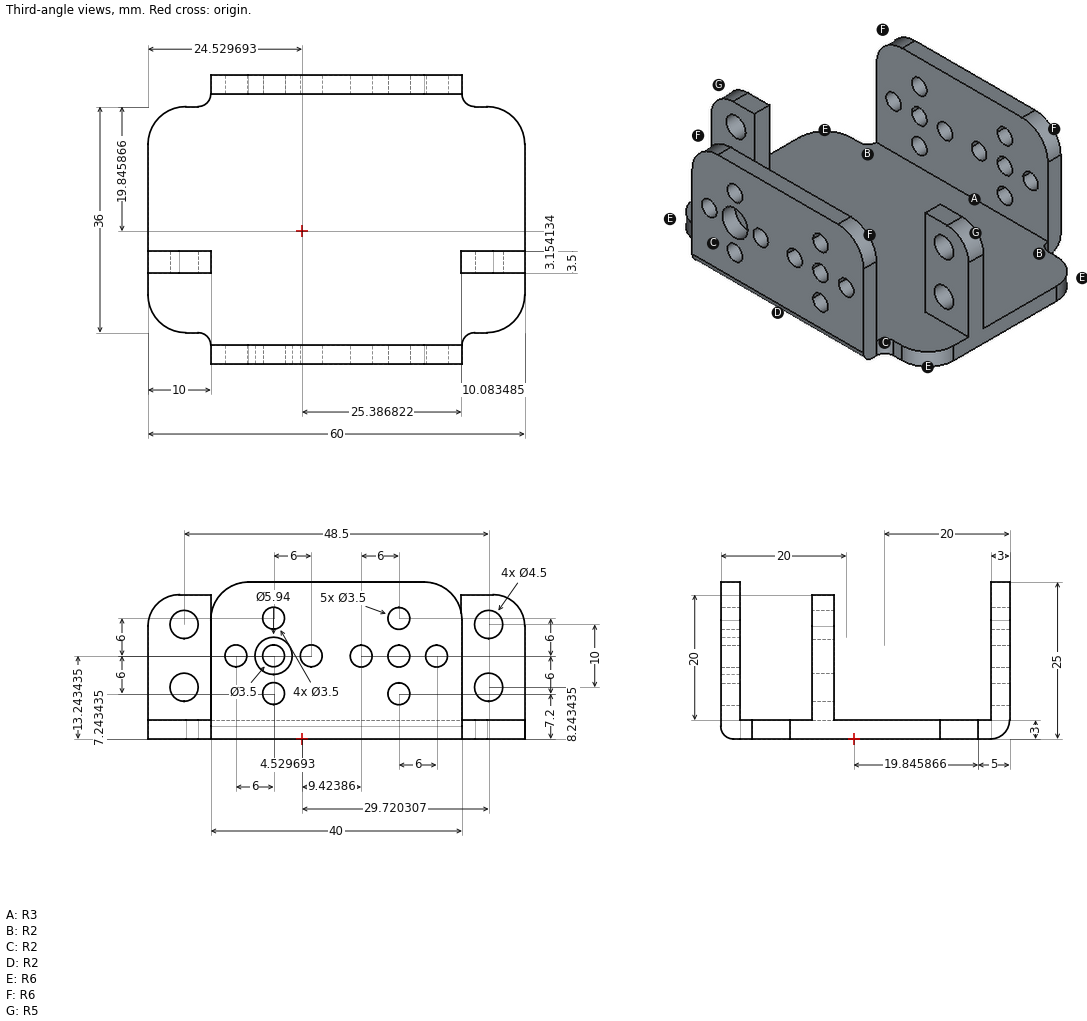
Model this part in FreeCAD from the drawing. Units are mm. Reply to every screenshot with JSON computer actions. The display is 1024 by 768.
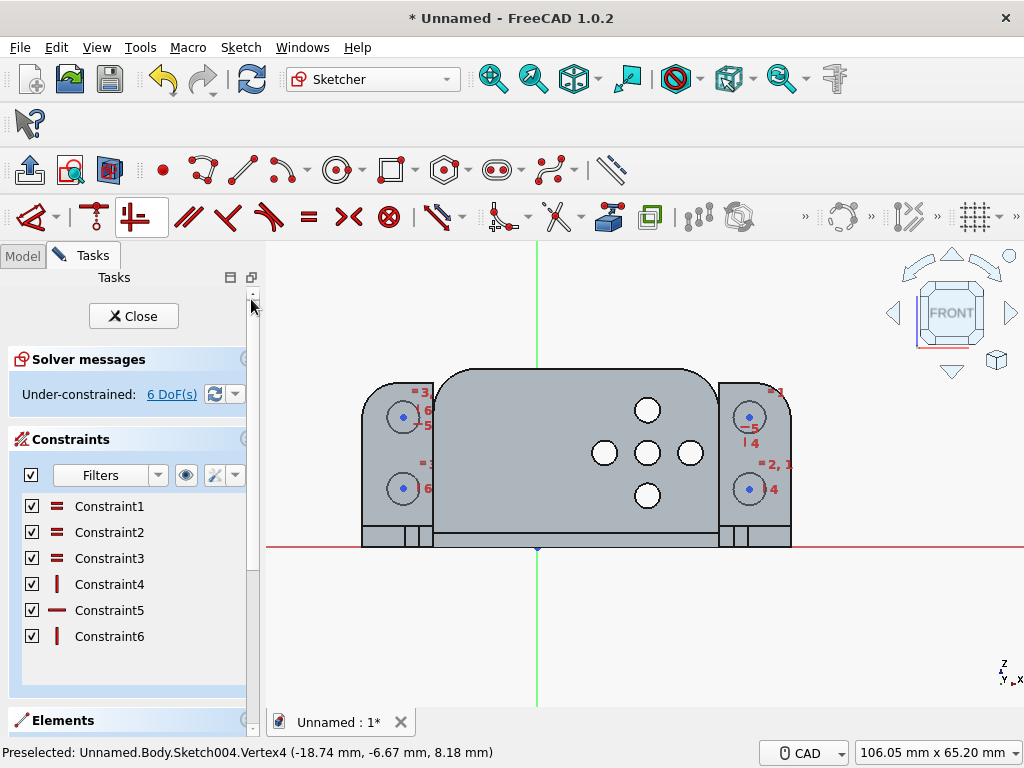
{"action": "left_click", "coordinate": [750, 489]}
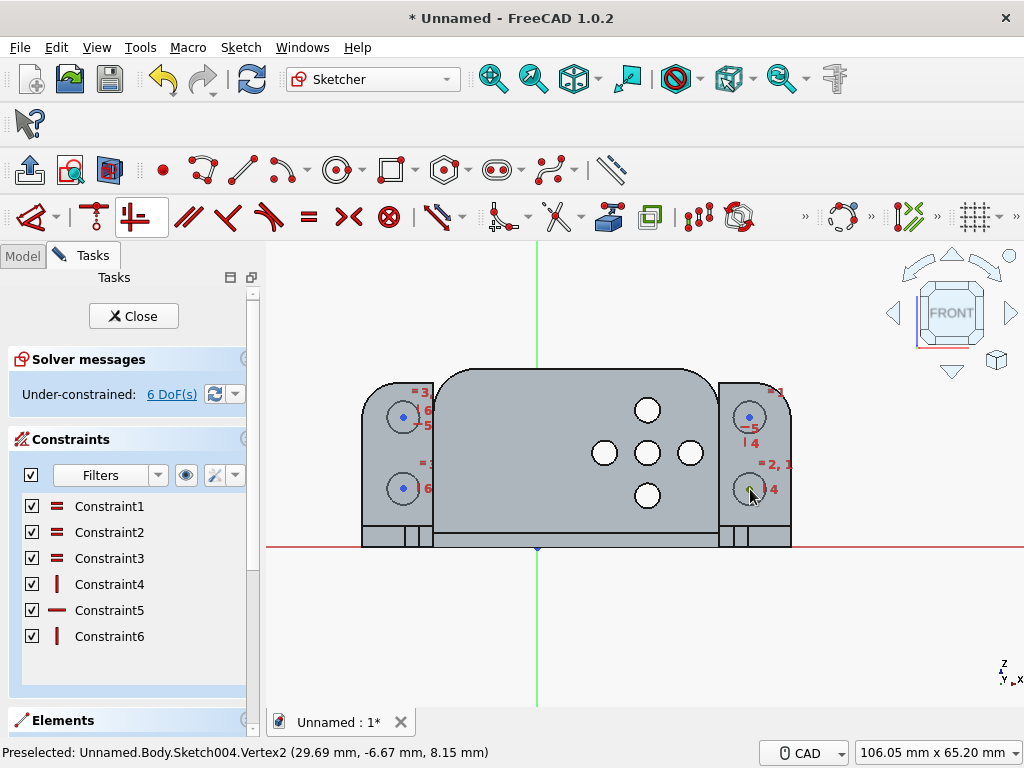
{"action": "left_click", "coordinate": [403, 489]}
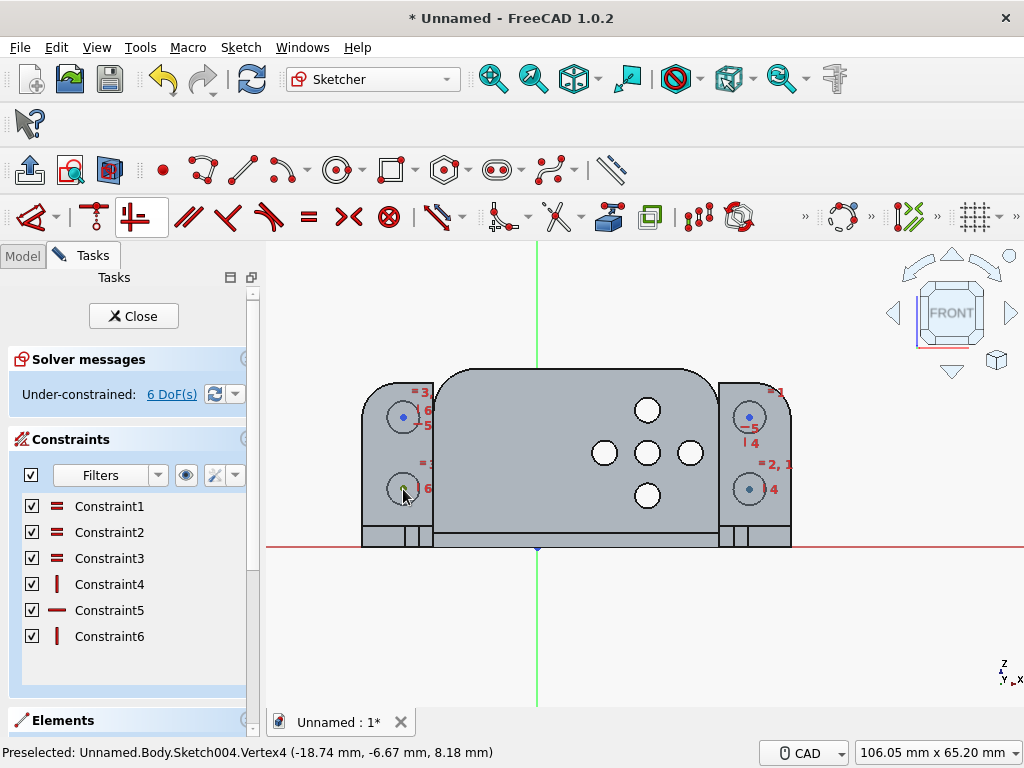
{"action": "left_click", "coordinate": [162, 218]}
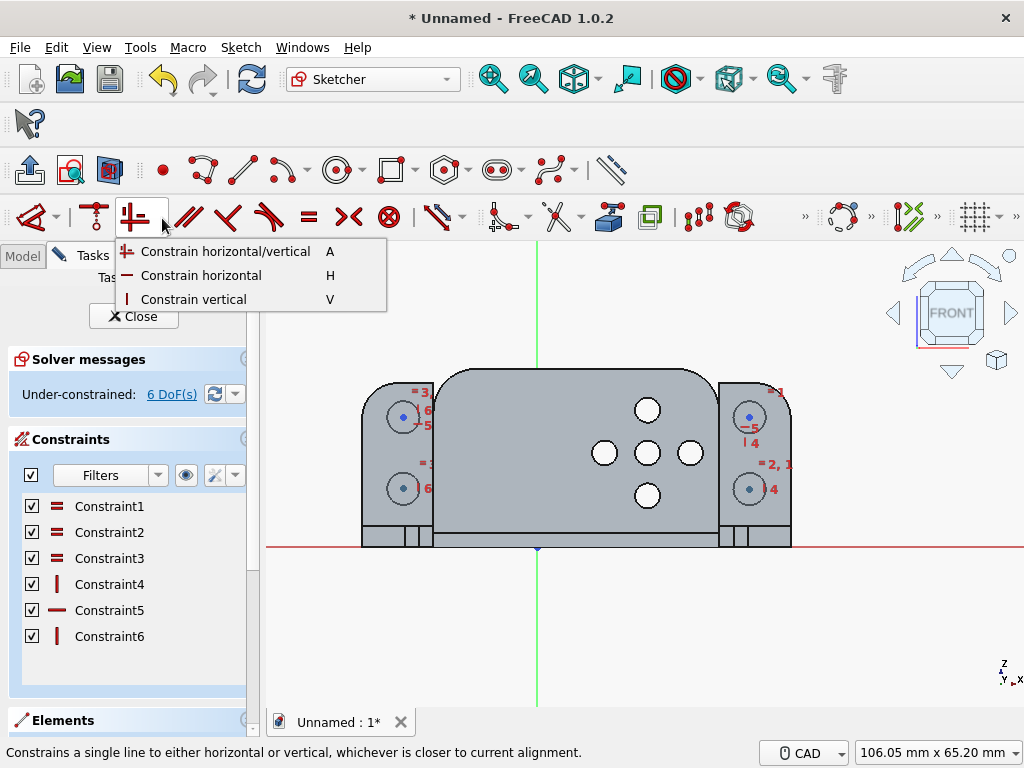
{"action": "left_click", "coordinate": [251, 275]}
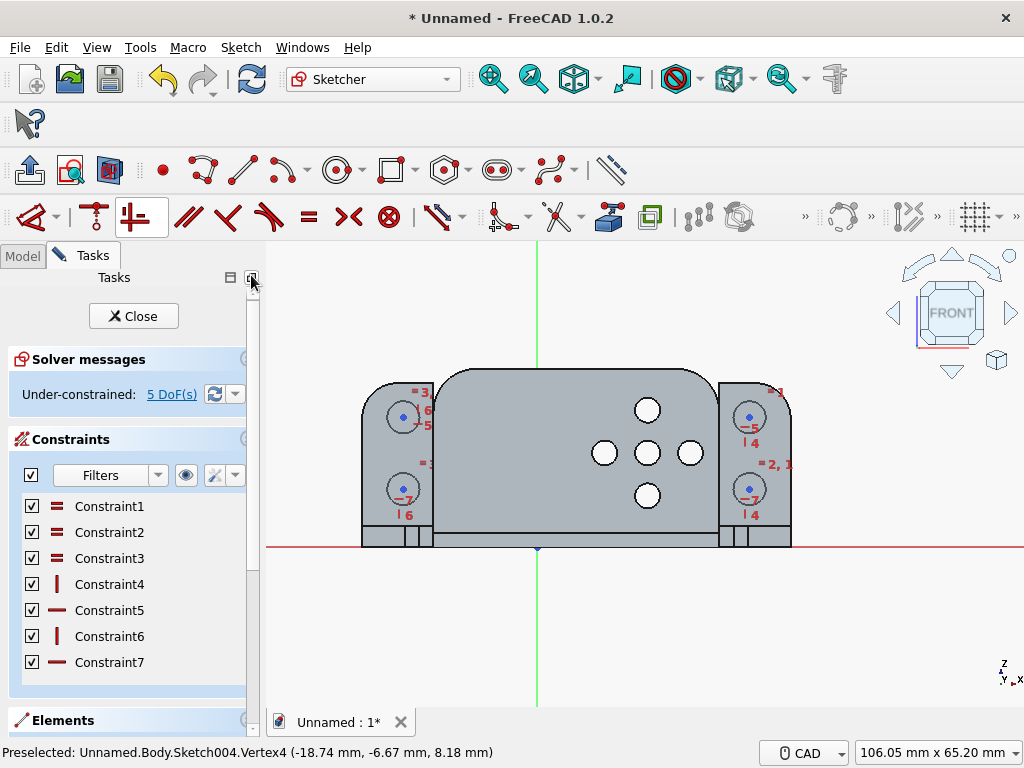
{"action": "left_click", "coordinate": [32, 218]}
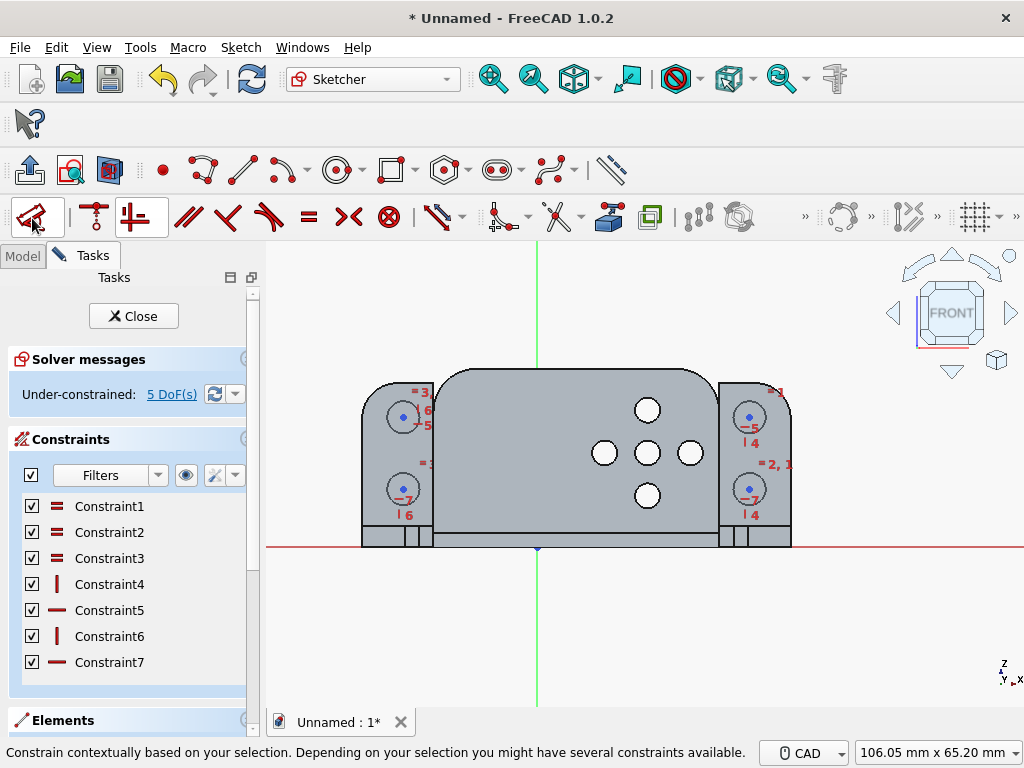
{"action": "scroll", "coordinate": [761, 406], "scroll_direction": "up", "scroll_amount": 2}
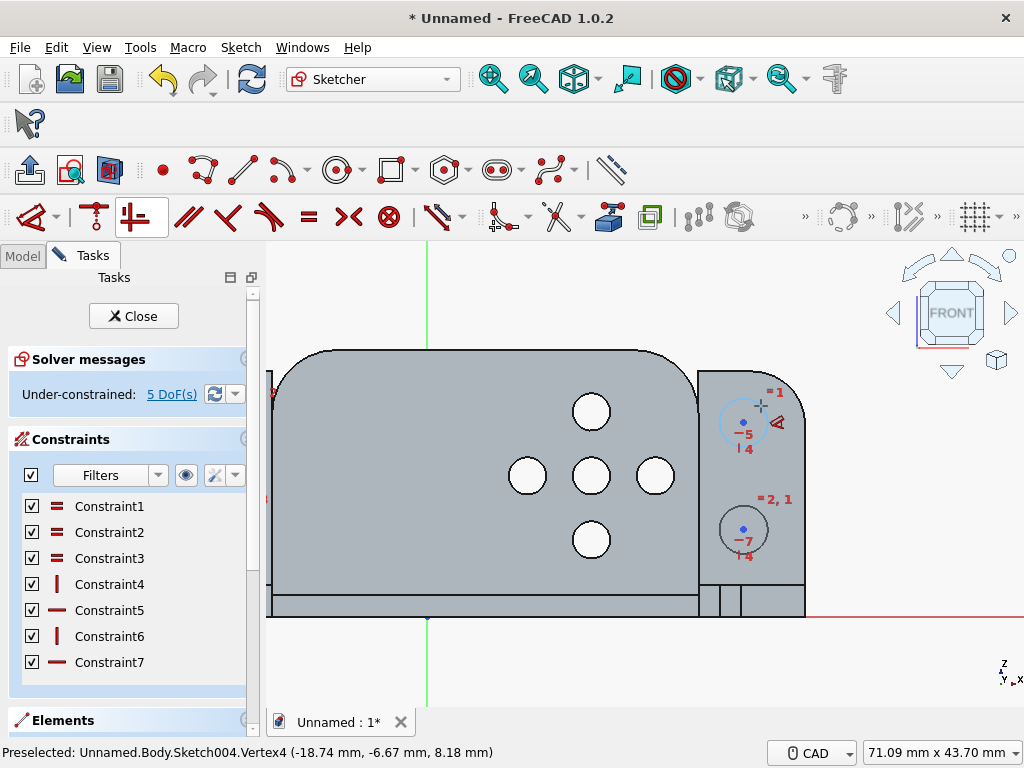
{"action": "left_click", "coordinate": [761, 406]}
{"action": "left_click", "coordinate": [784, 384]}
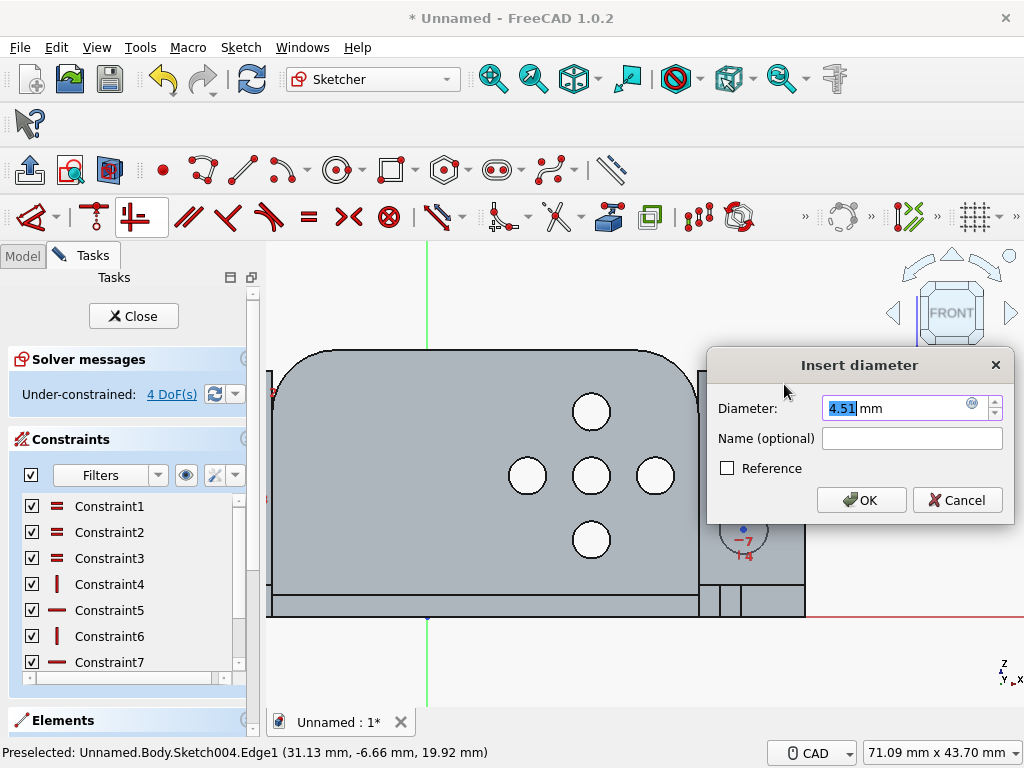
{"action": "type", "text": "4.5"}
{"action": "key", "text": "Return"}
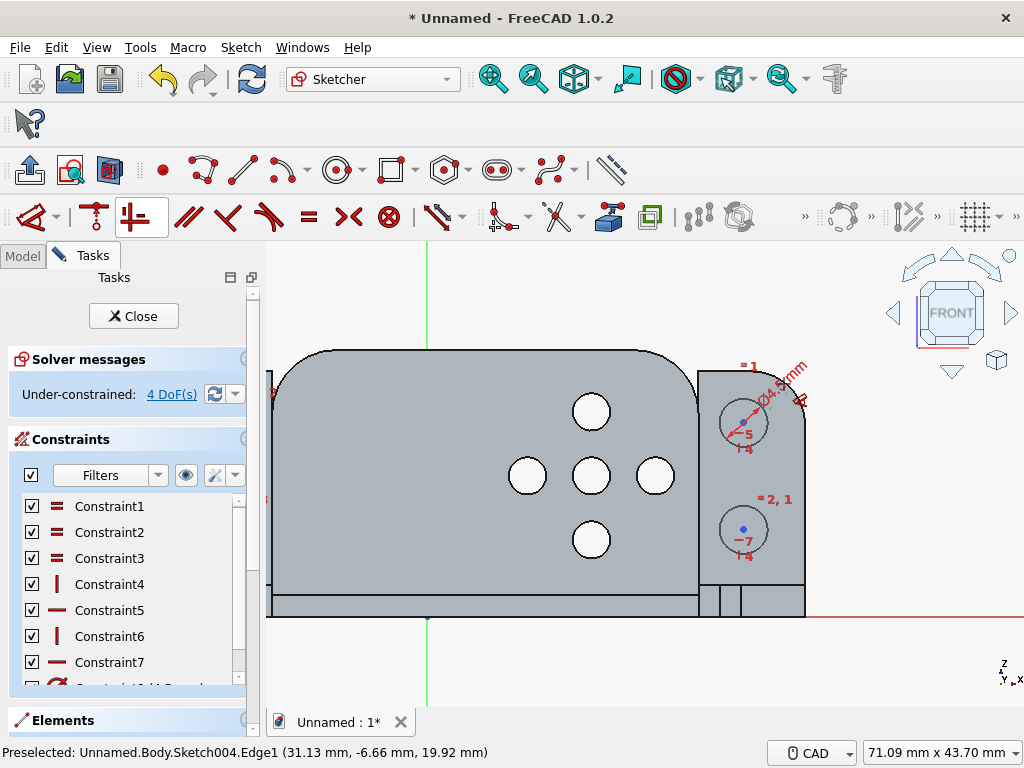
{"action": "left_click", "coordinate": [744, 423]}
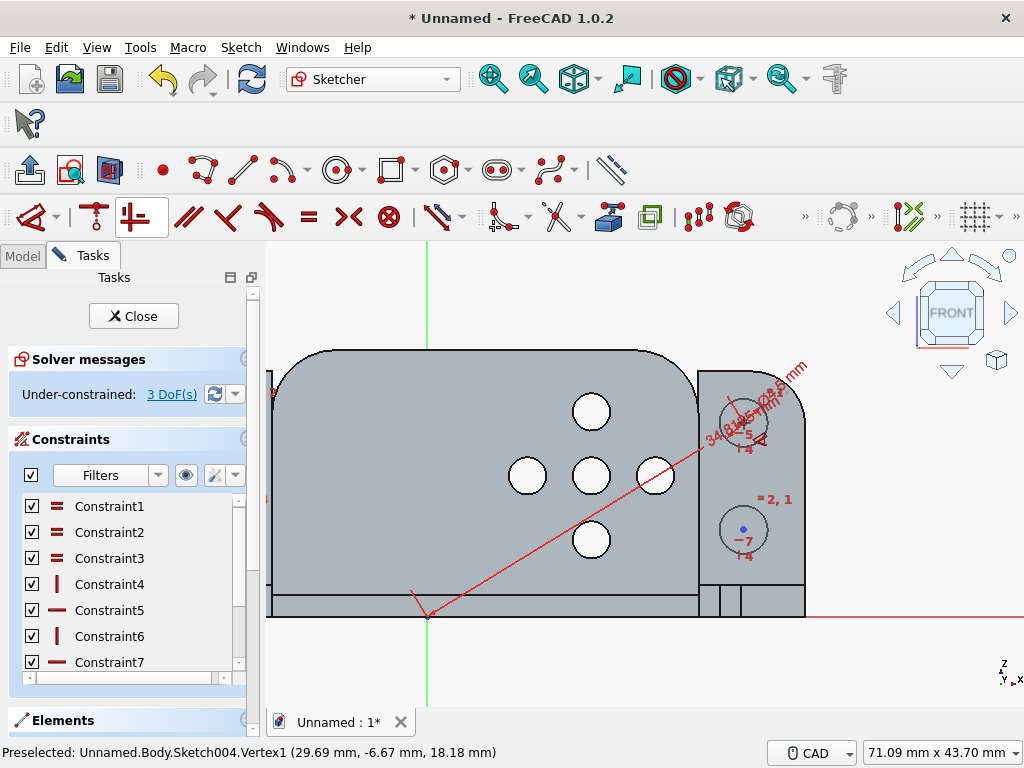
{"action": "left_click", "coordinate": [744, 530]}
{"action": "left_click", "coordinate": [778, 476]}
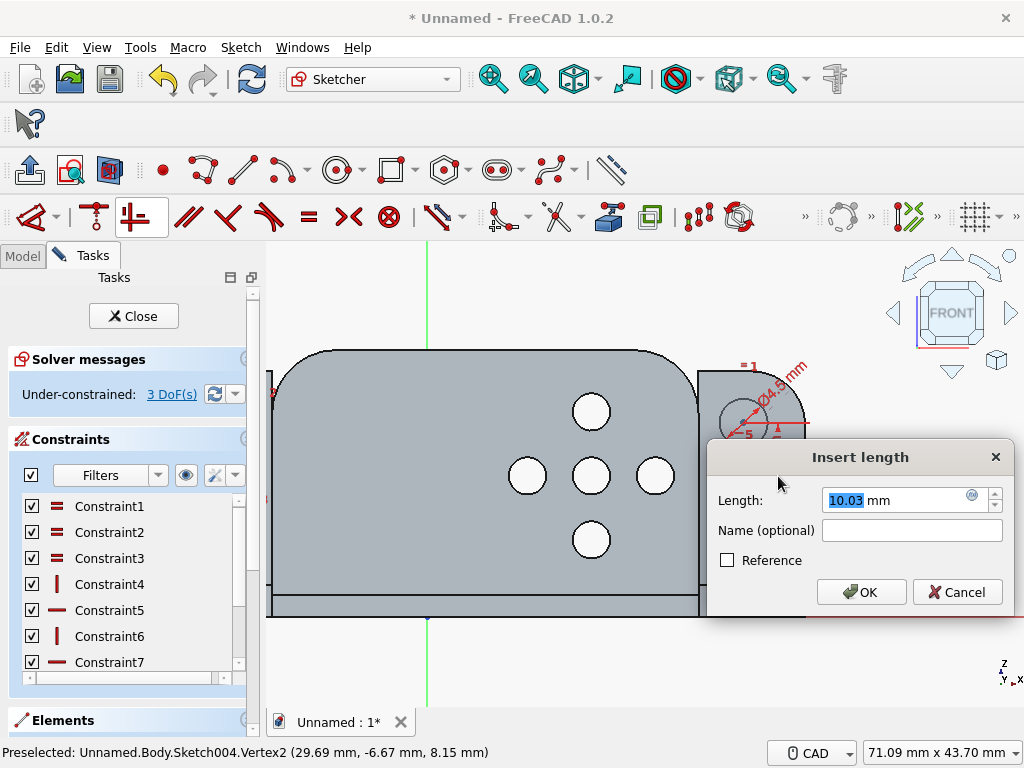
{"action": "type", "text": "10"}
{"action": "key", "text": "Return"}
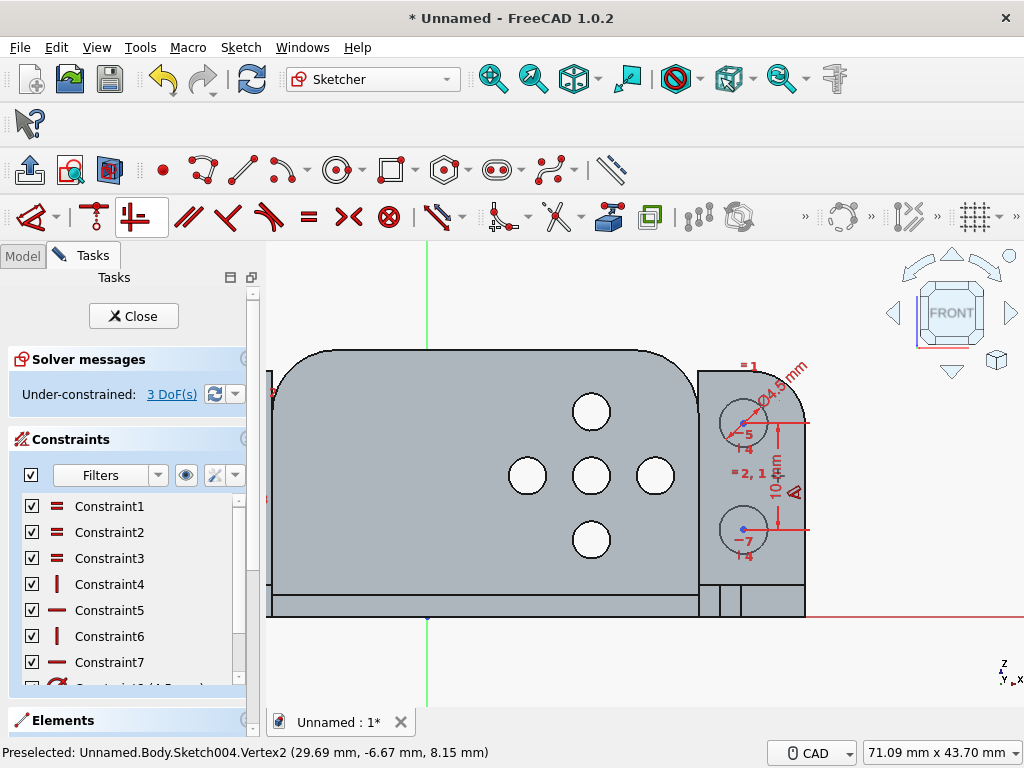
{"action": "left_click", "coordinate": [744, 423]}